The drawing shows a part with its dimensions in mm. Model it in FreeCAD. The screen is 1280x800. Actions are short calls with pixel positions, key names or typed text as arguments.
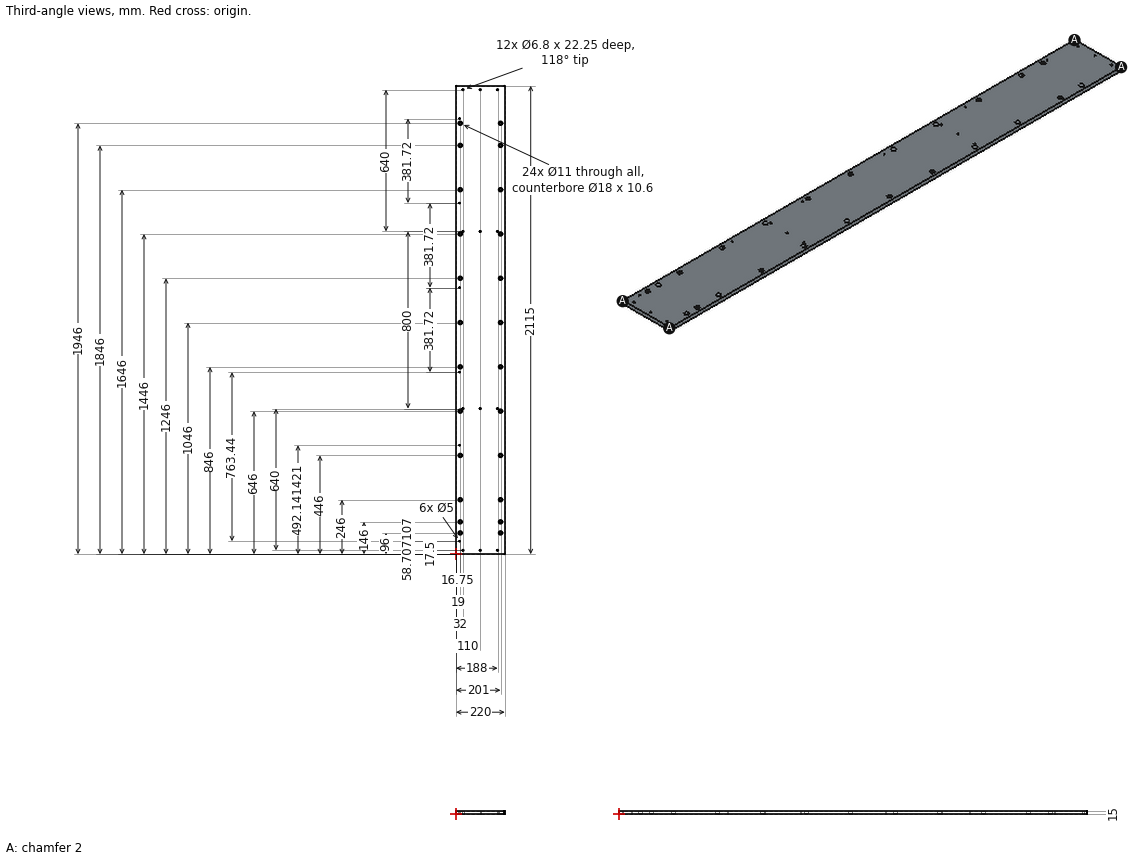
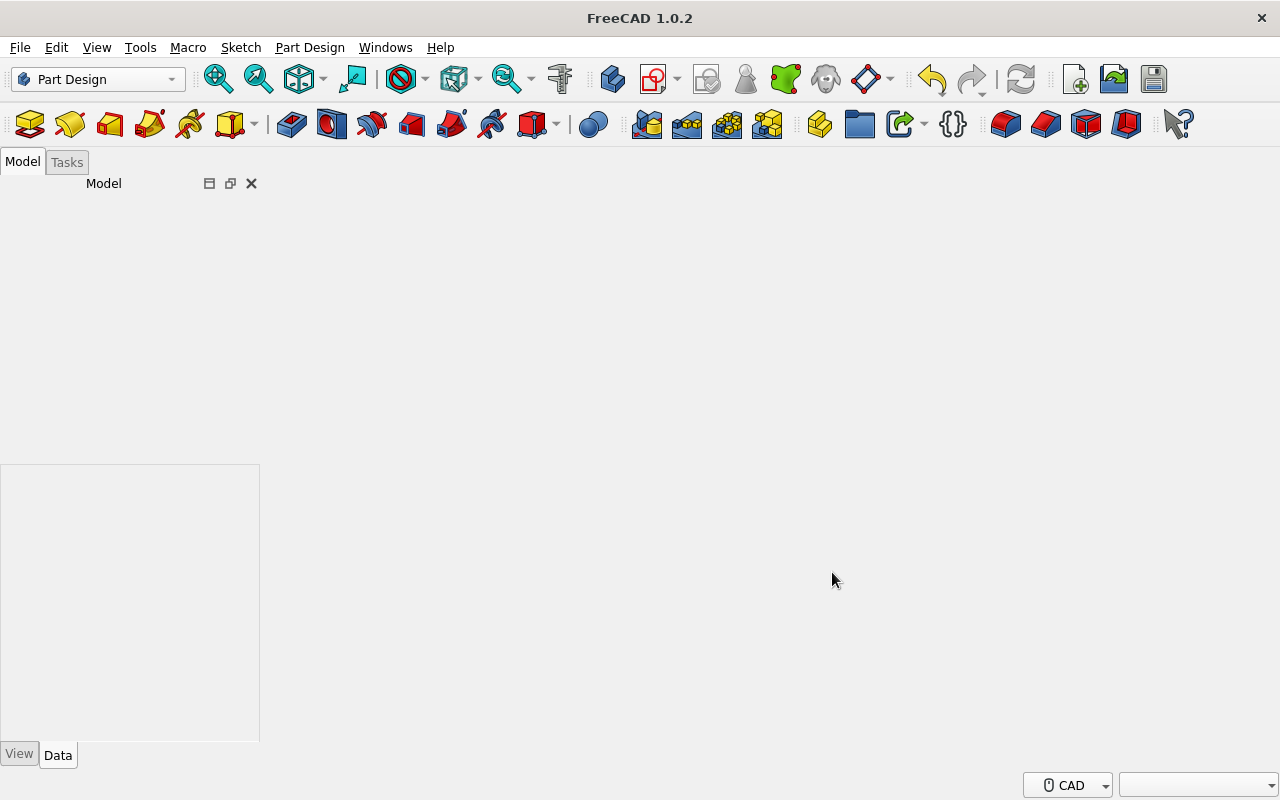
click(1074, 80)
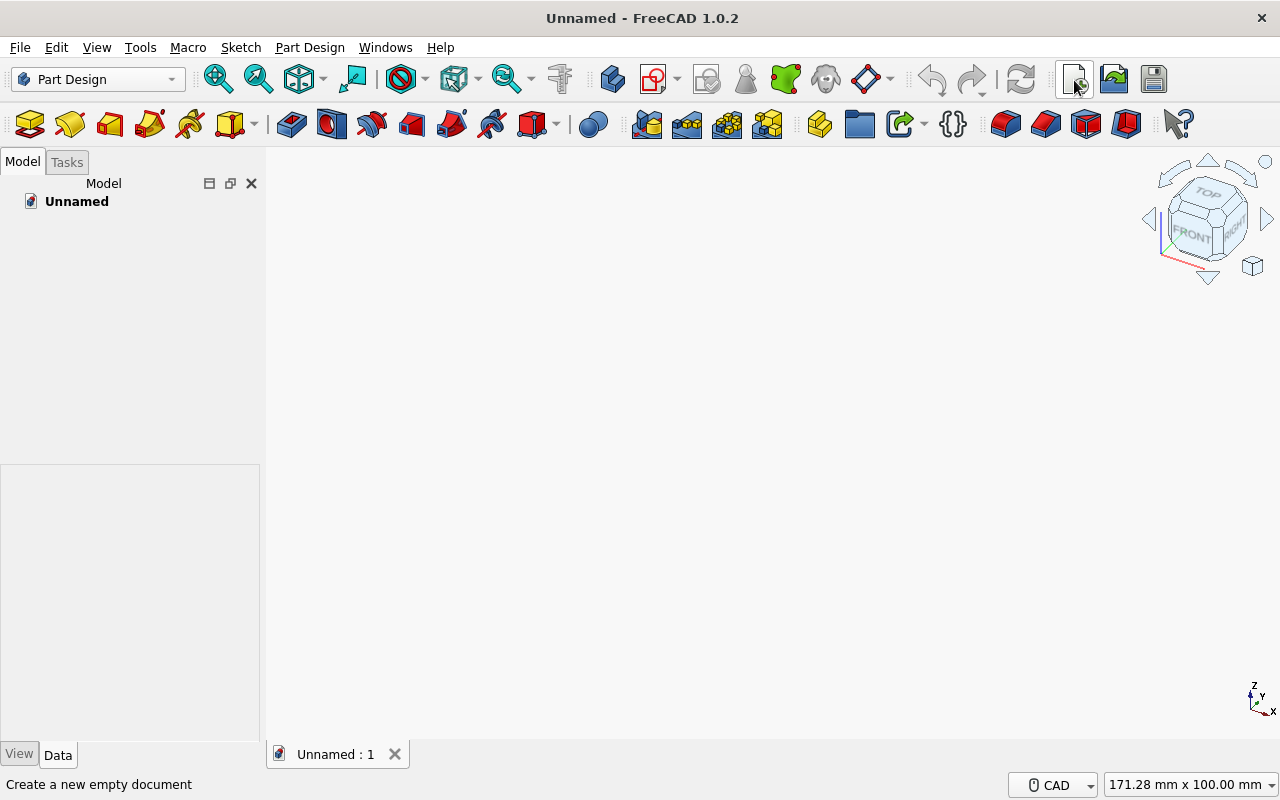
click(654, 80)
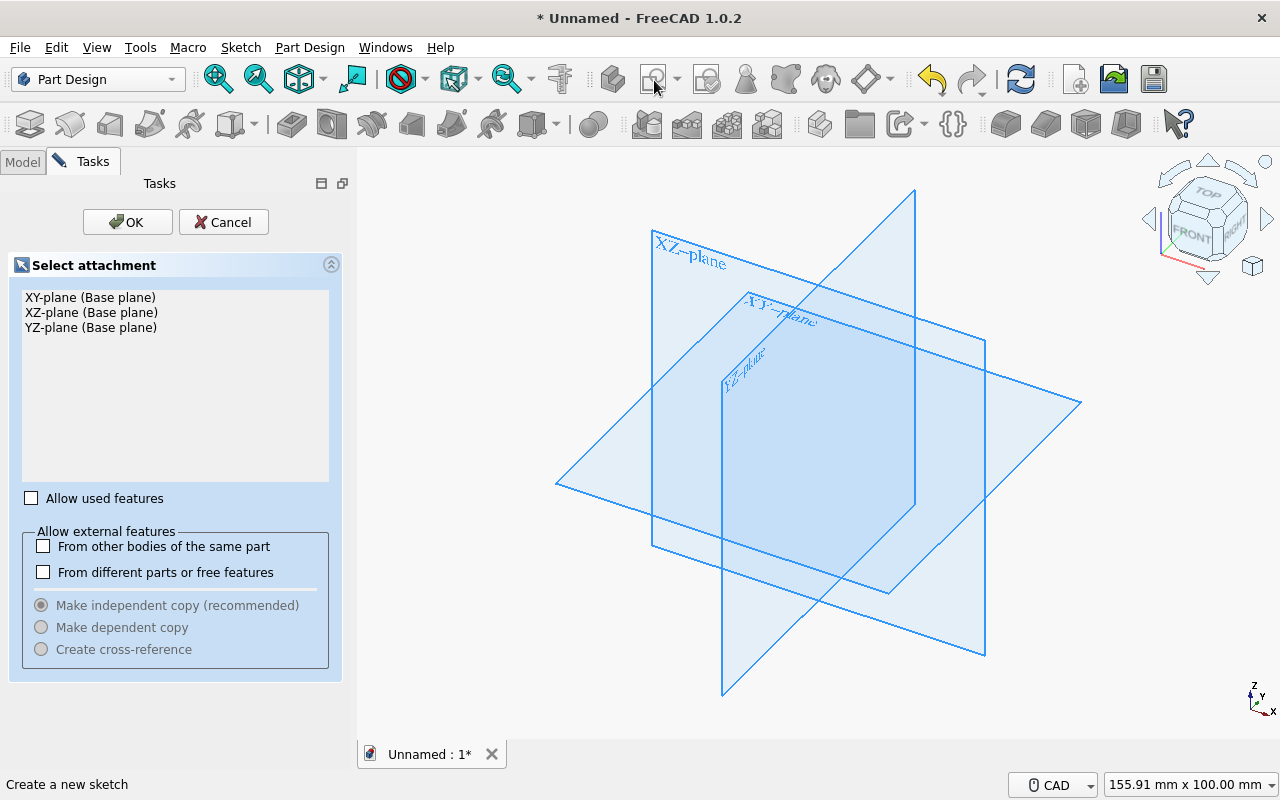
click(82, 298)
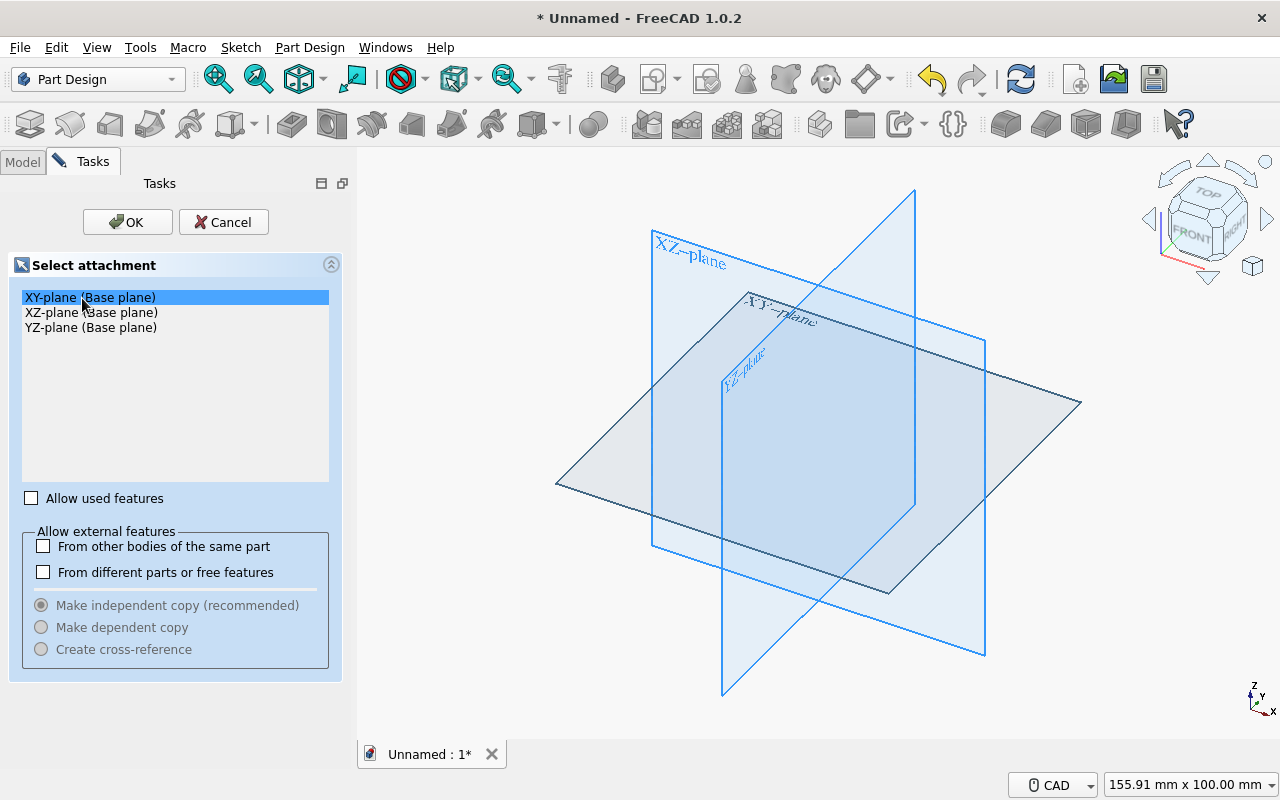
click(128, 222)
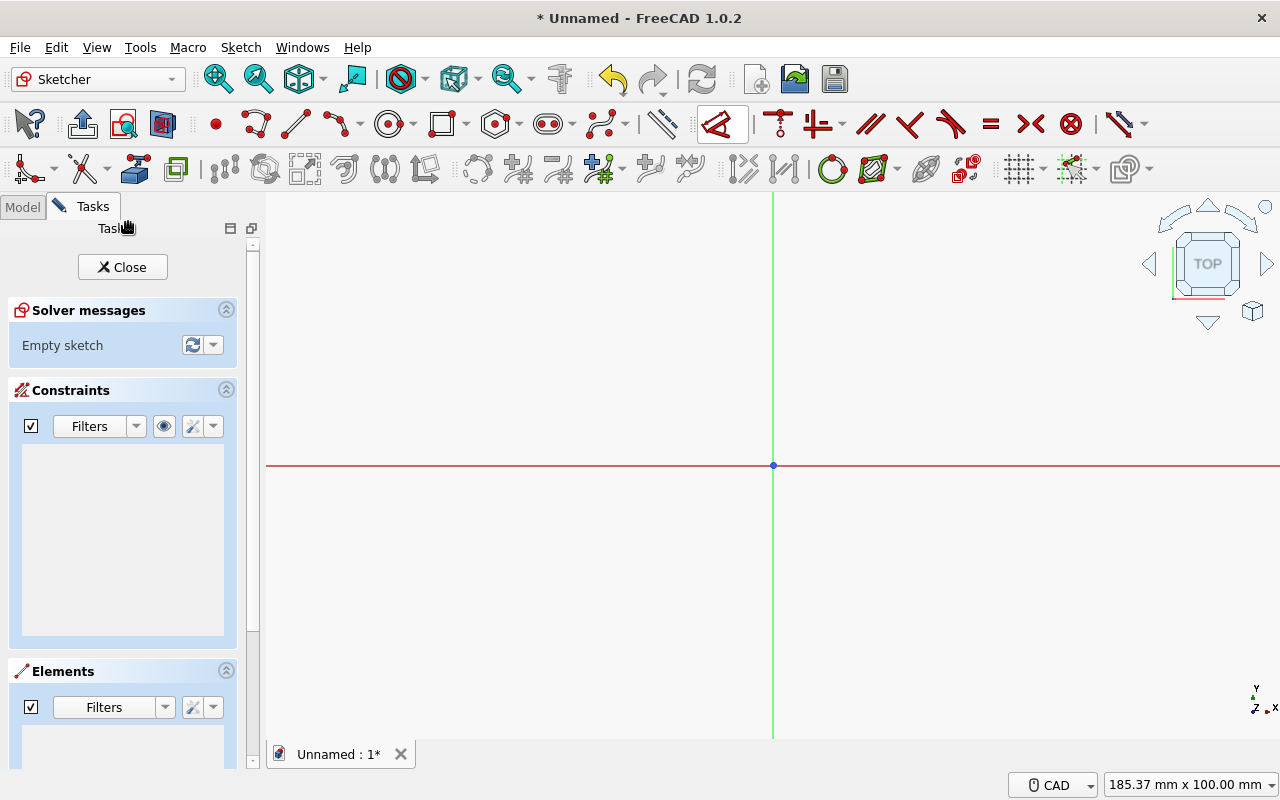
scroll(681, 665, down, 17)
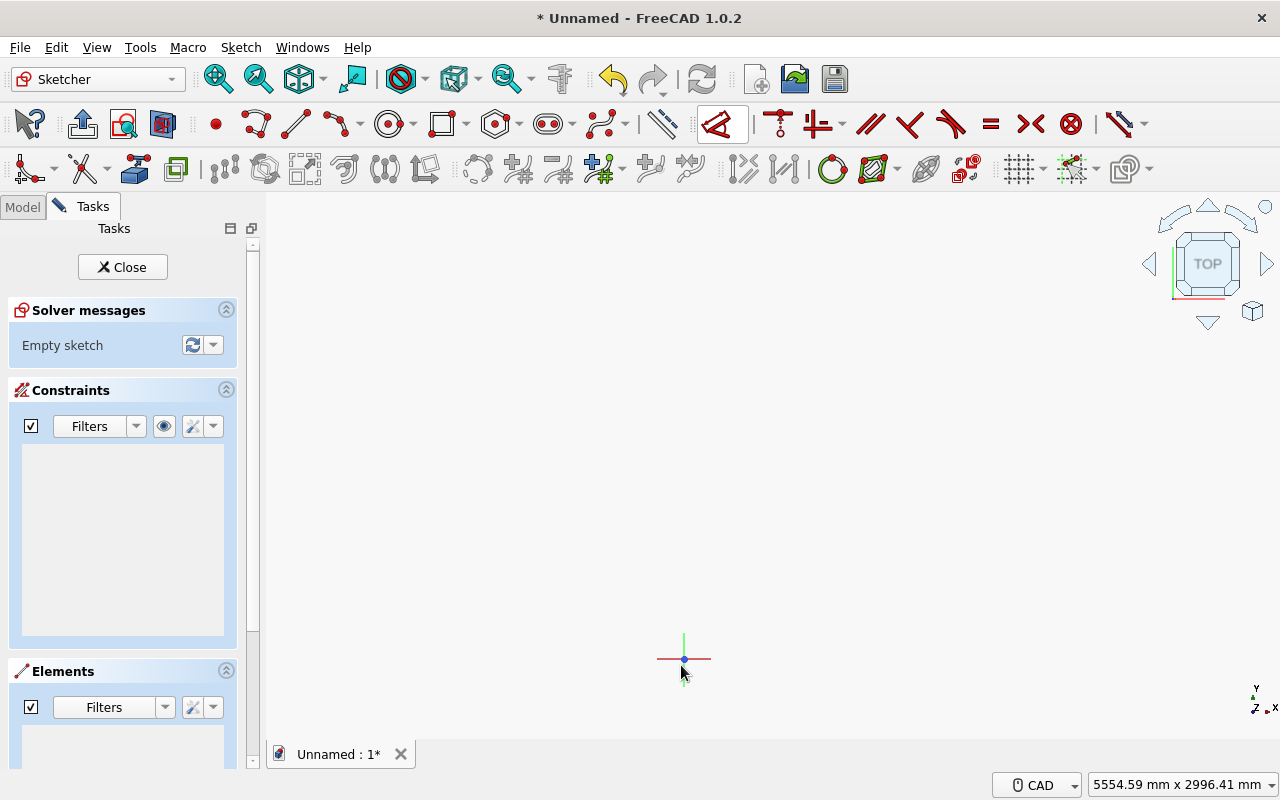
click(442, 124)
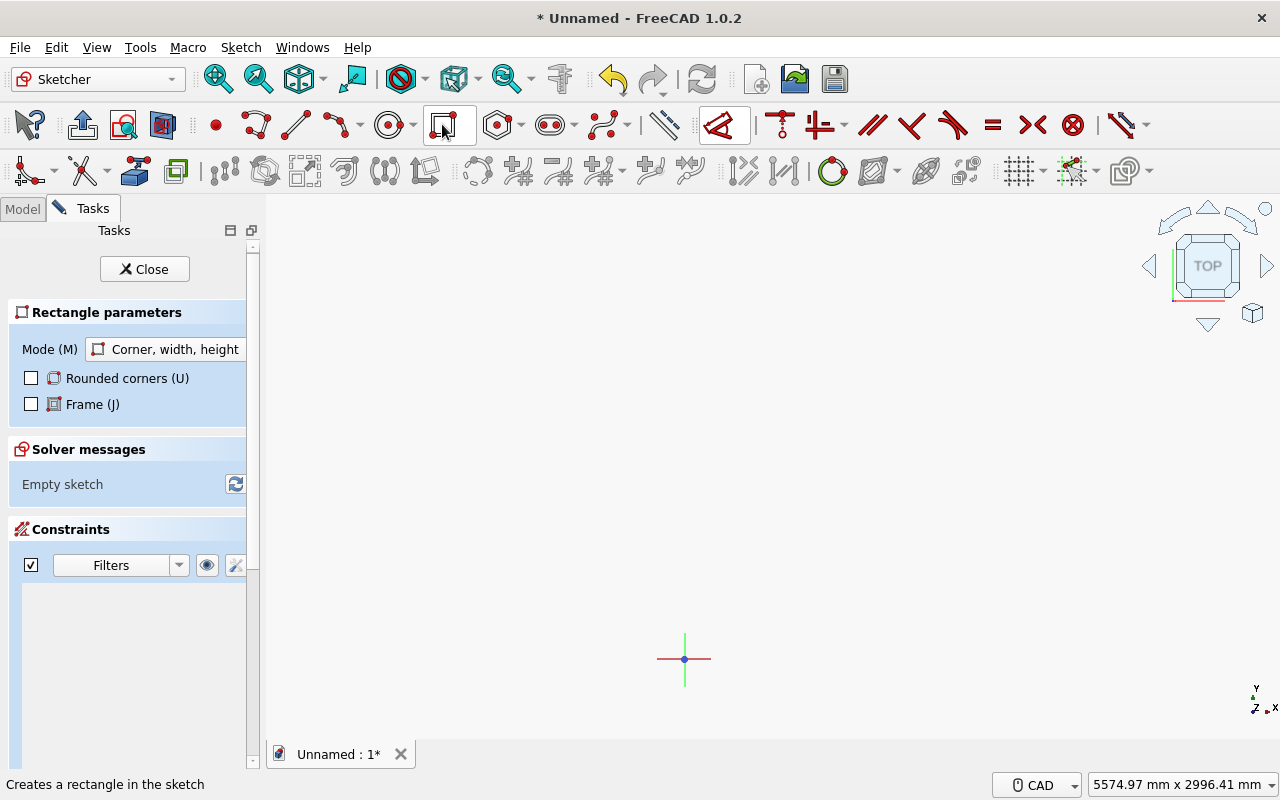
click(685, 659)
move(725, 275)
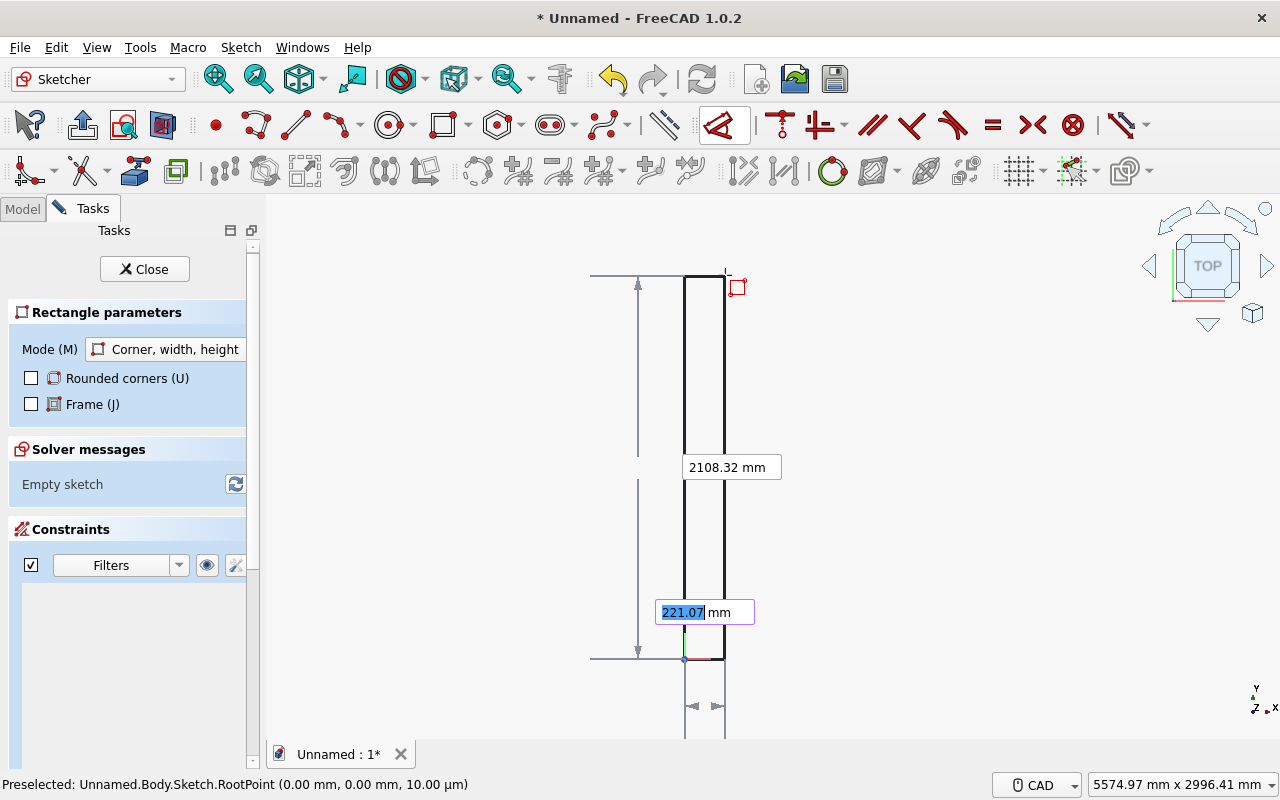
text(220)
key(Tab)
text(2115)
key(Return)
key(Escape)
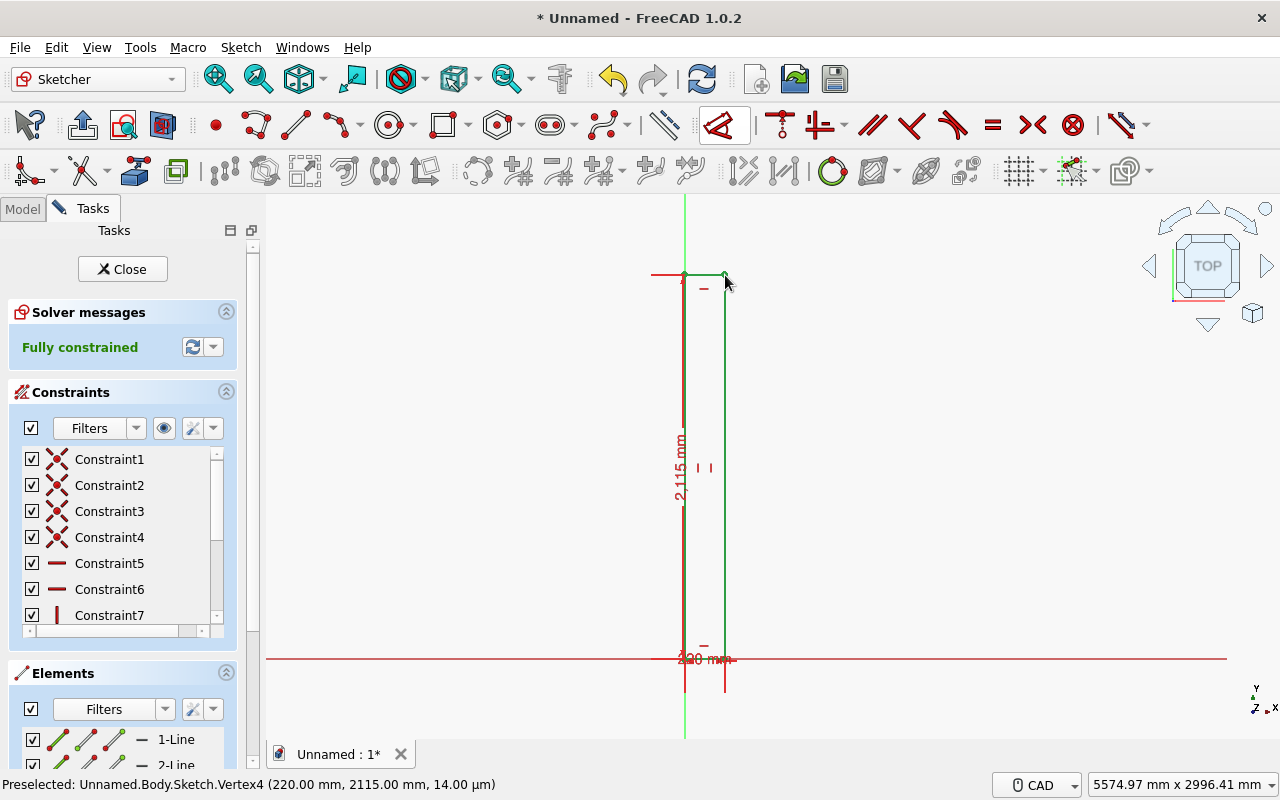
click(123, 269)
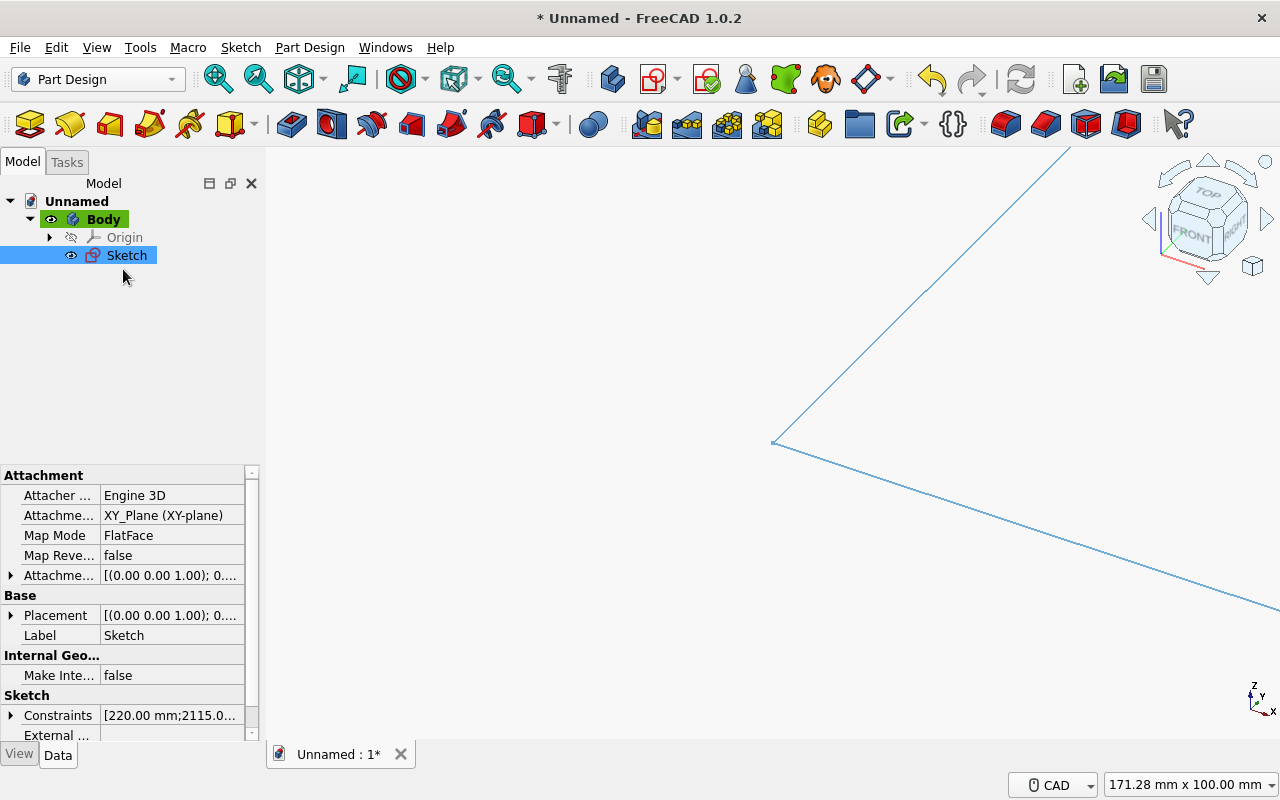
click(30, 124)